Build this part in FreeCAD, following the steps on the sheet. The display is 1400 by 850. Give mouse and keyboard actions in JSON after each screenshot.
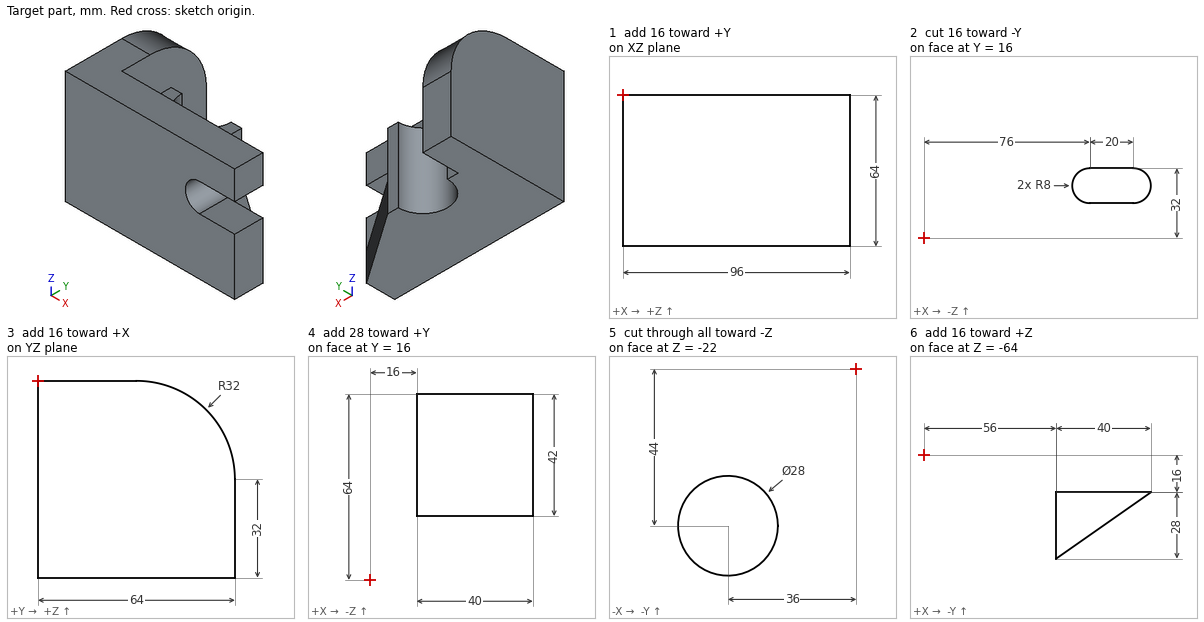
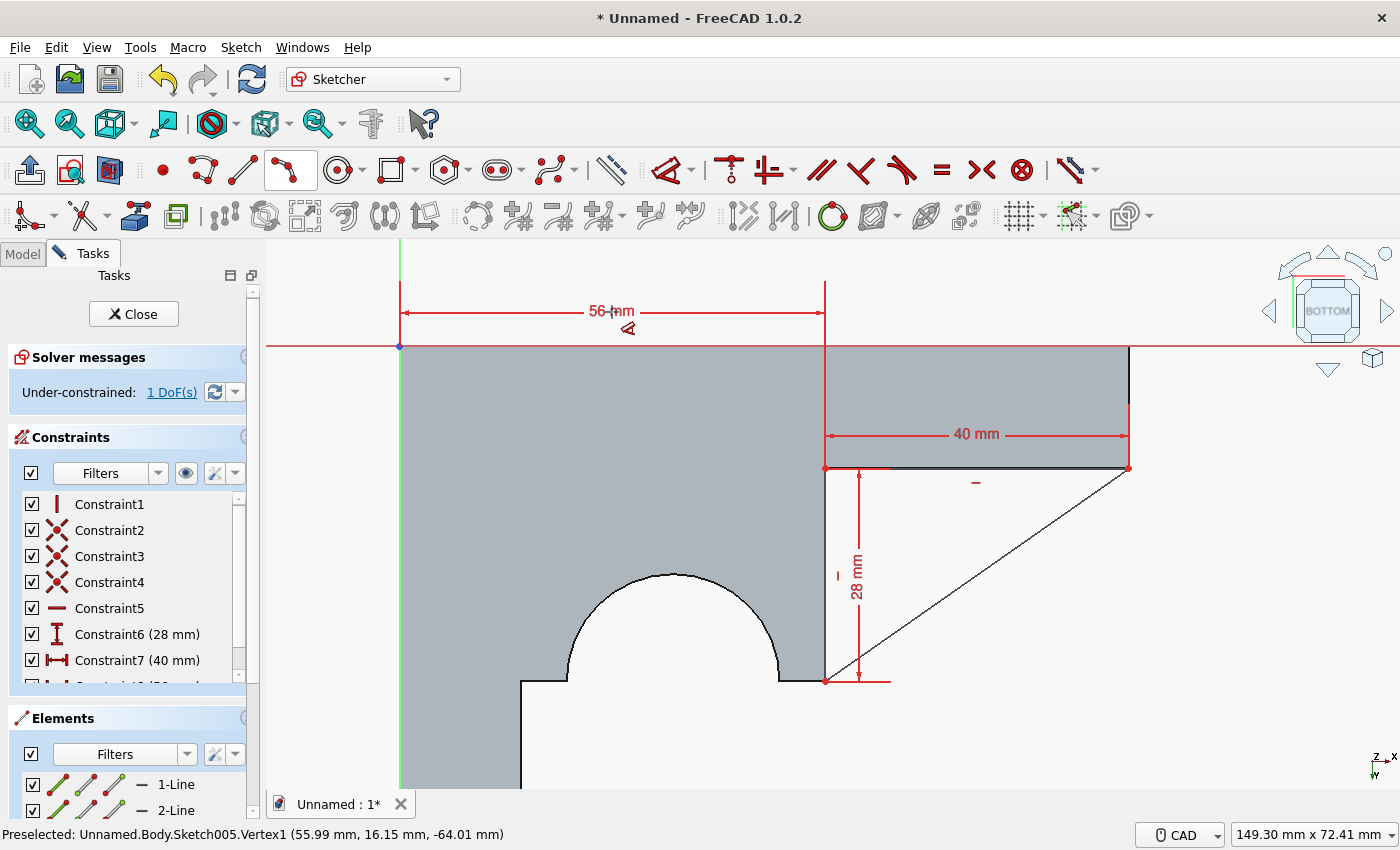
{"action": "left_click", "coordinate": [825, 469]}
{"action": "left_click", "coordinate": [366, 408]}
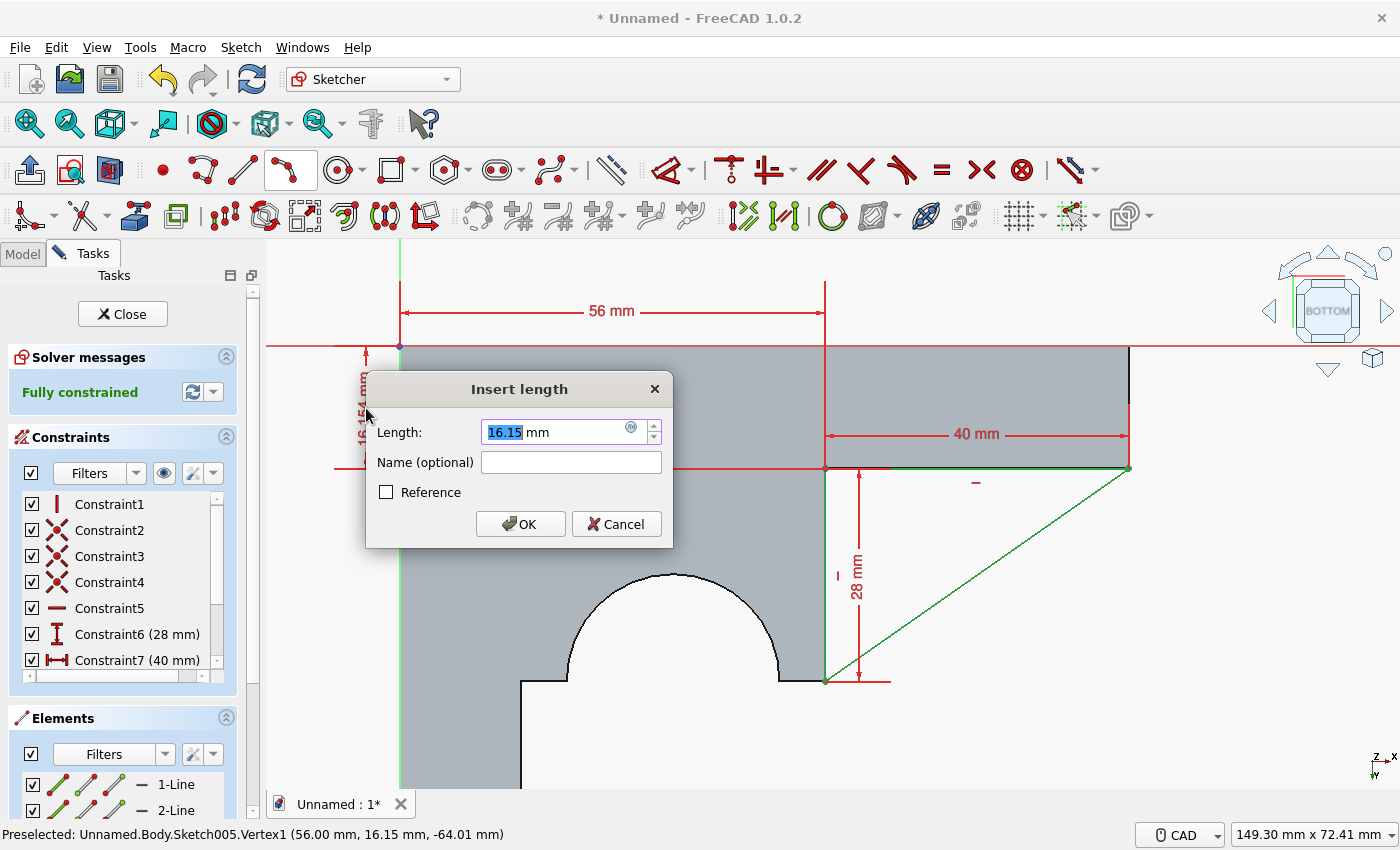
{"action": "type", "text": "16"}
{"action": "key", "text": "Return"}
{"action": "key", "text": "Escape"}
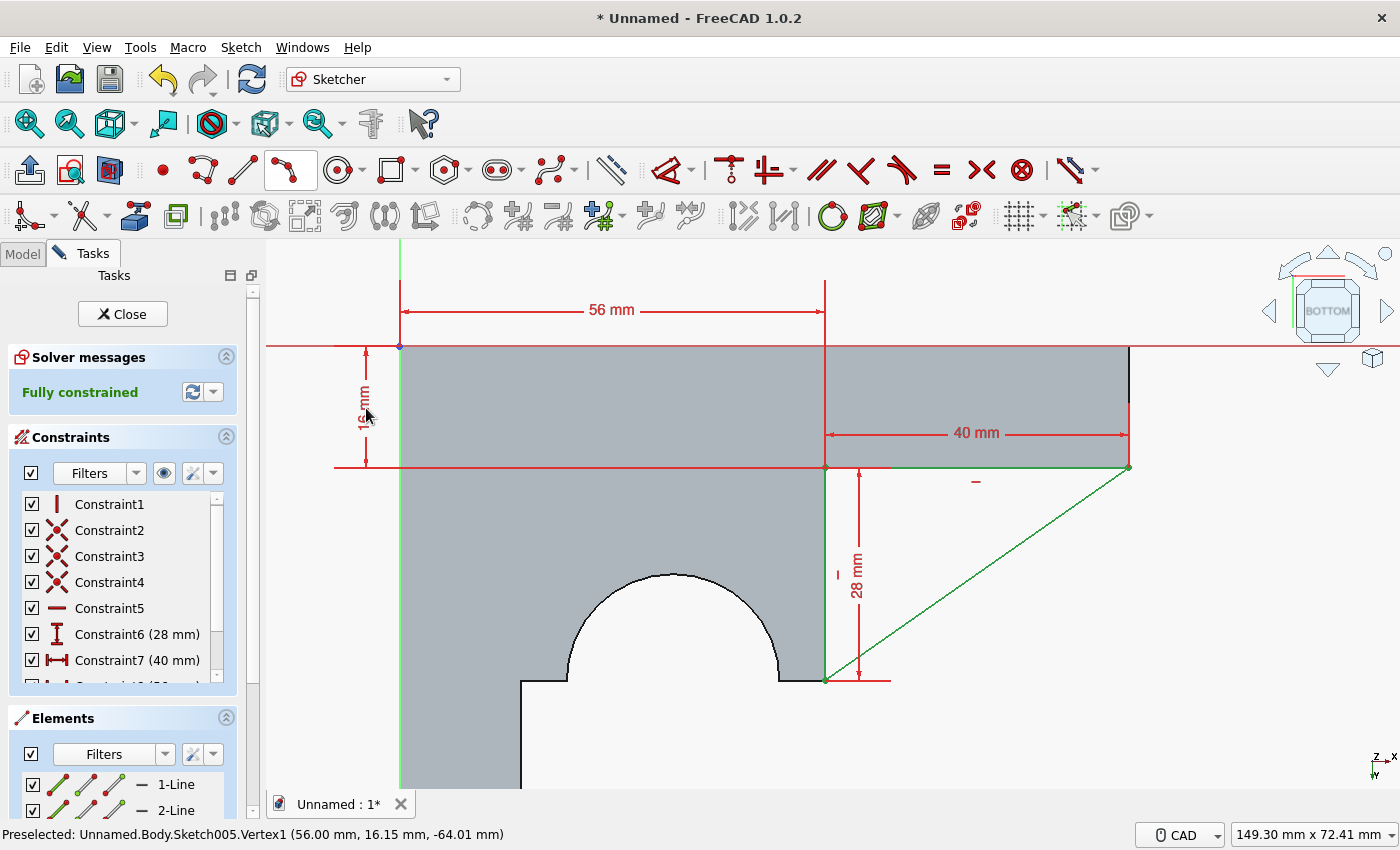
{"action": "left_click", "coordinate": [123, 314]}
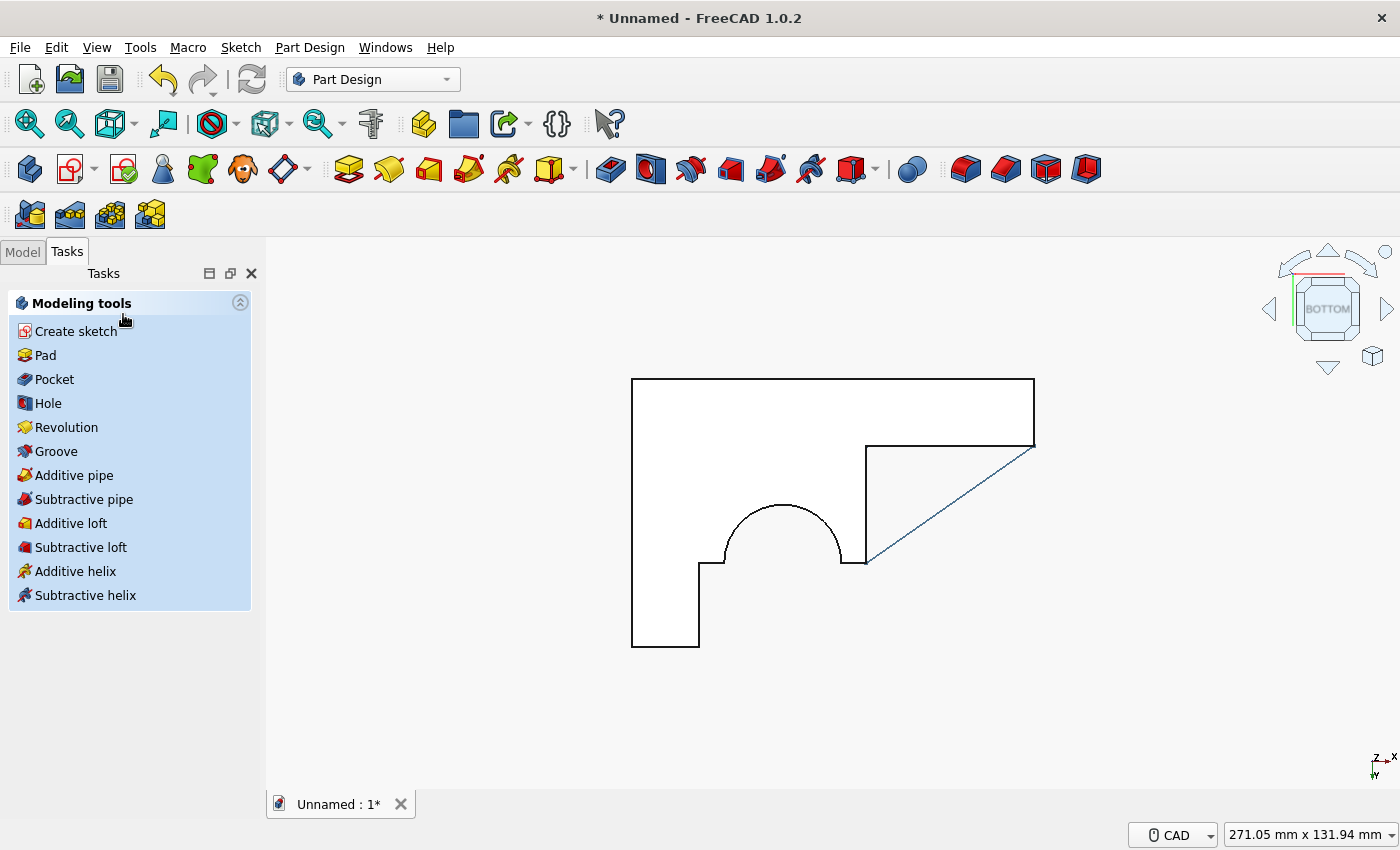
{"action": "left_click", "coordinate": [350, 170]}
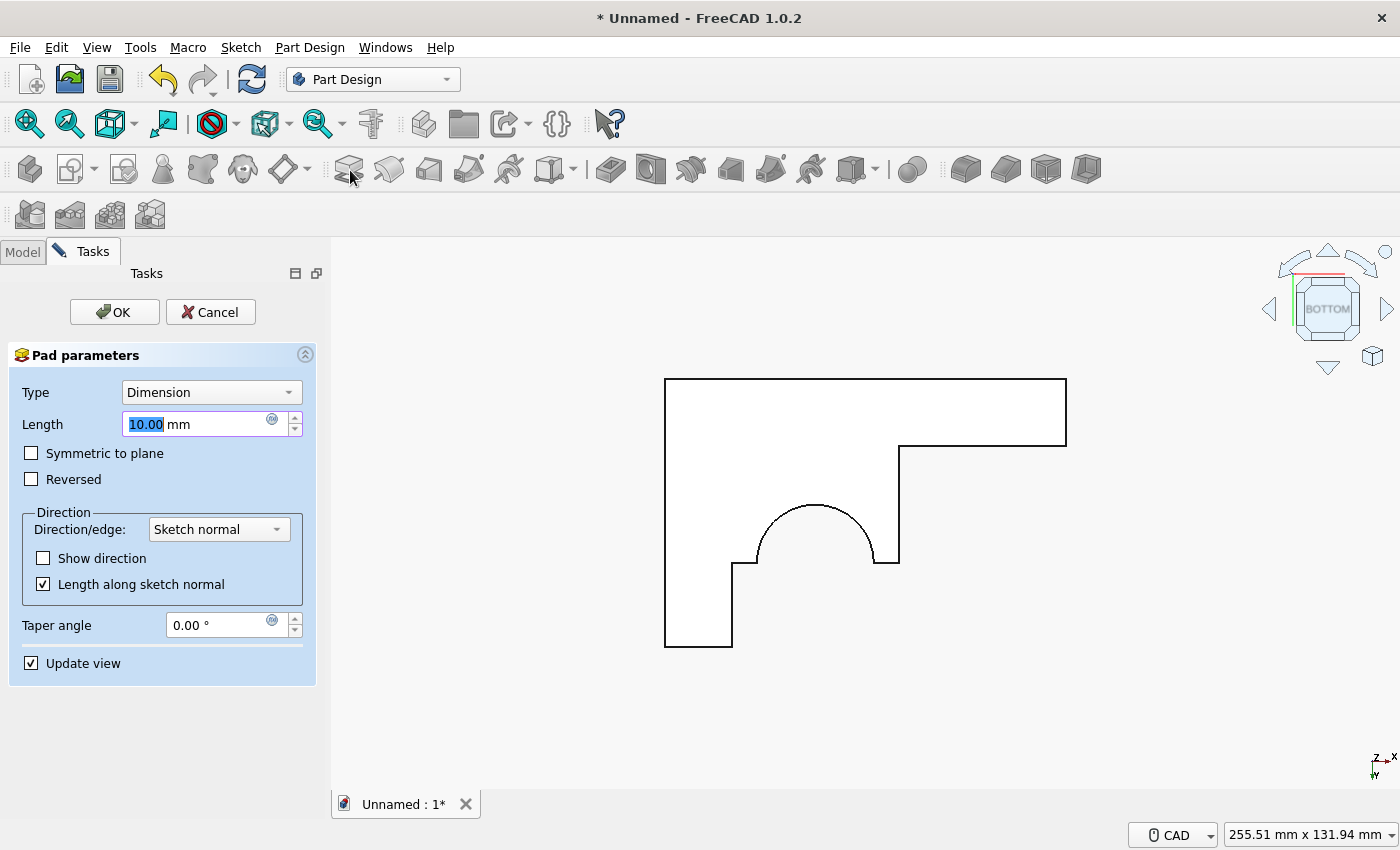
{"action": "type", "text": "16"}
{"action": "key", "text": "Tab"}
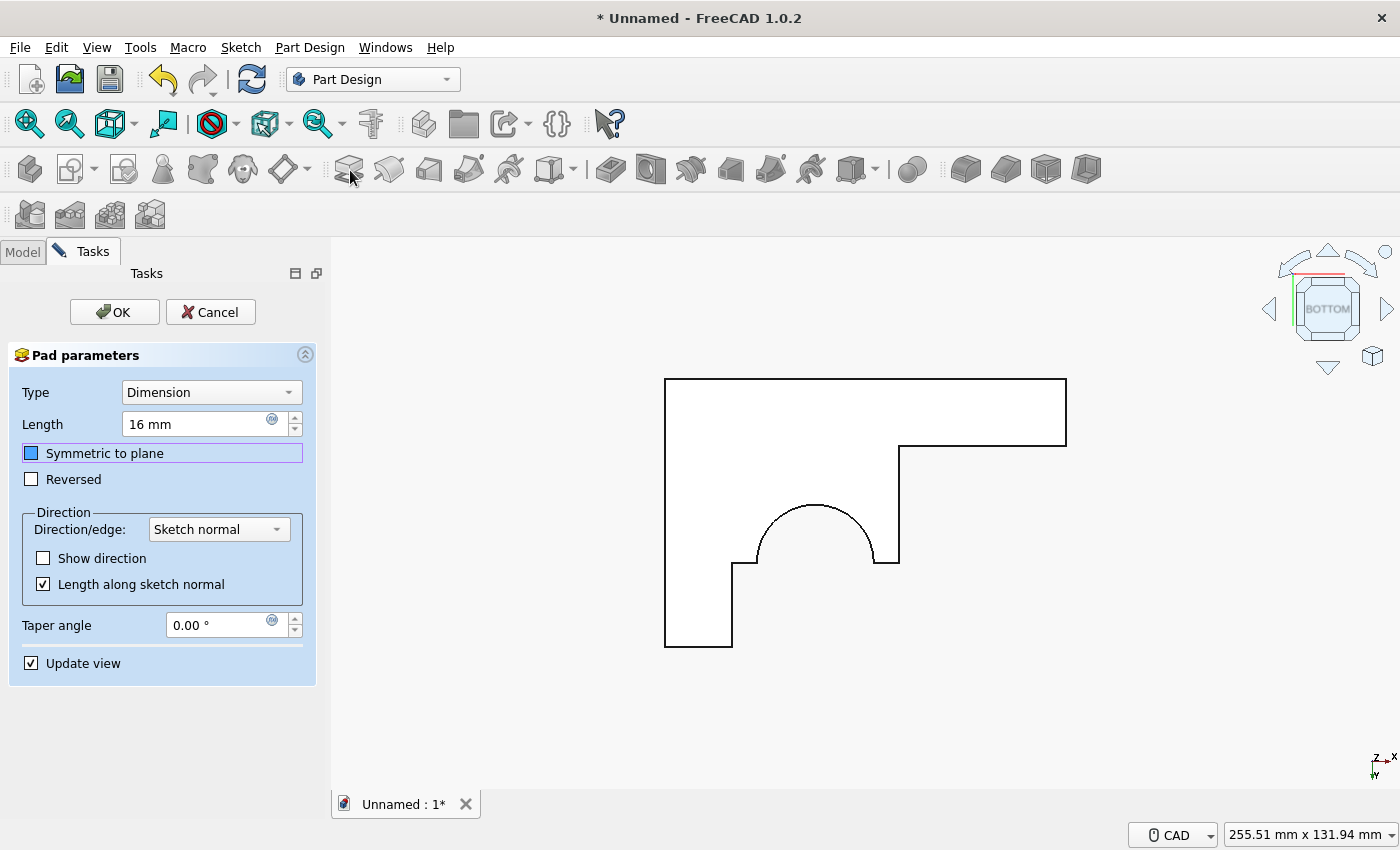
{"action": "left_click", "coordinate": [30, 479]}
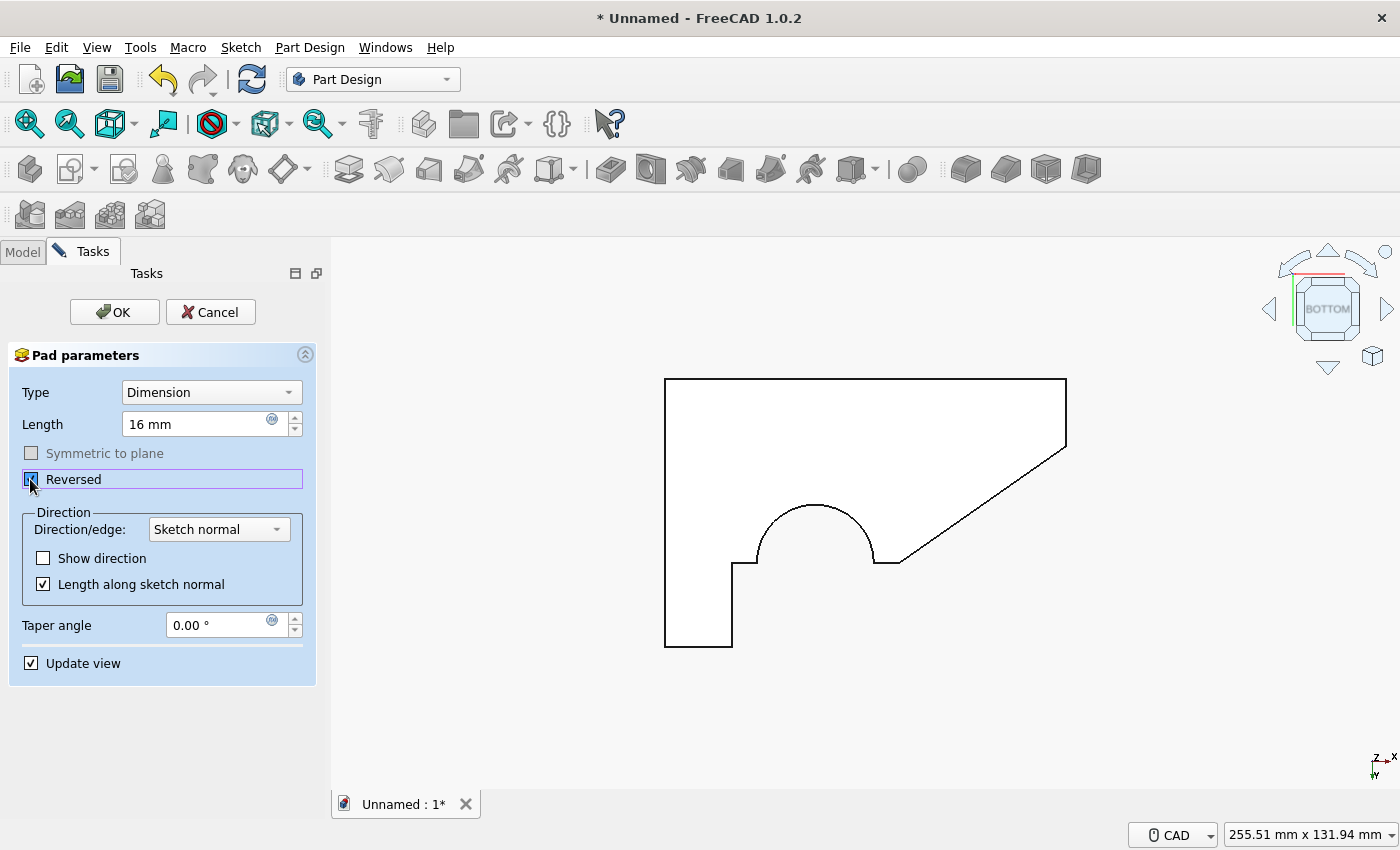
{"action": "left_click", "coordinate": [115, 312]}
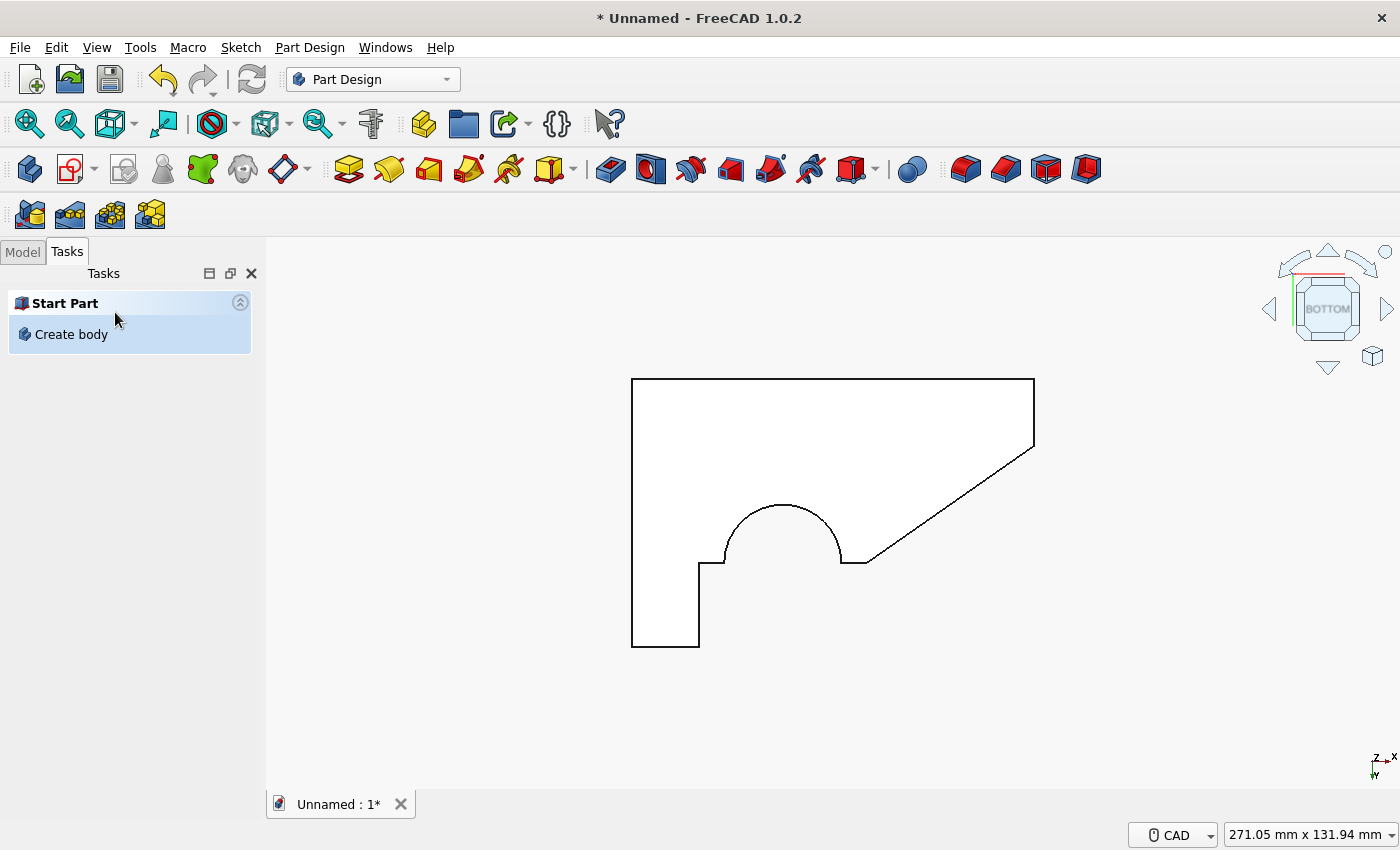
{"action": "key", "text": "0"}